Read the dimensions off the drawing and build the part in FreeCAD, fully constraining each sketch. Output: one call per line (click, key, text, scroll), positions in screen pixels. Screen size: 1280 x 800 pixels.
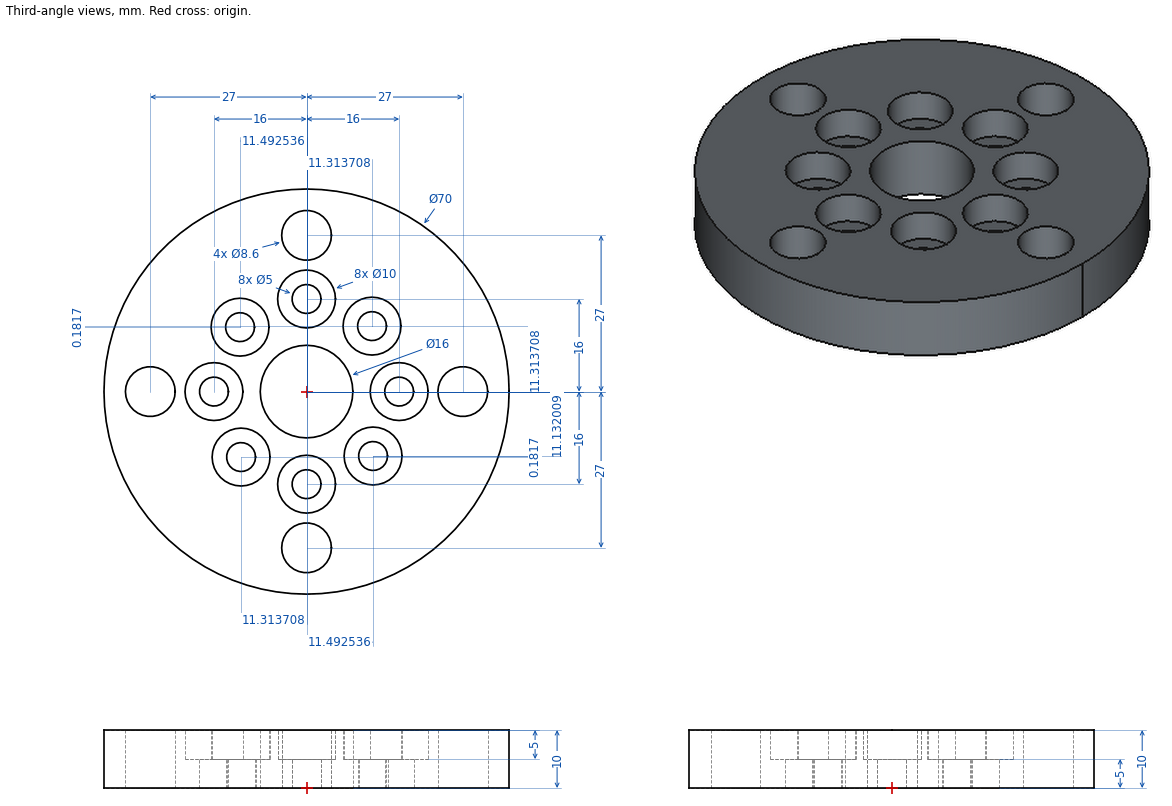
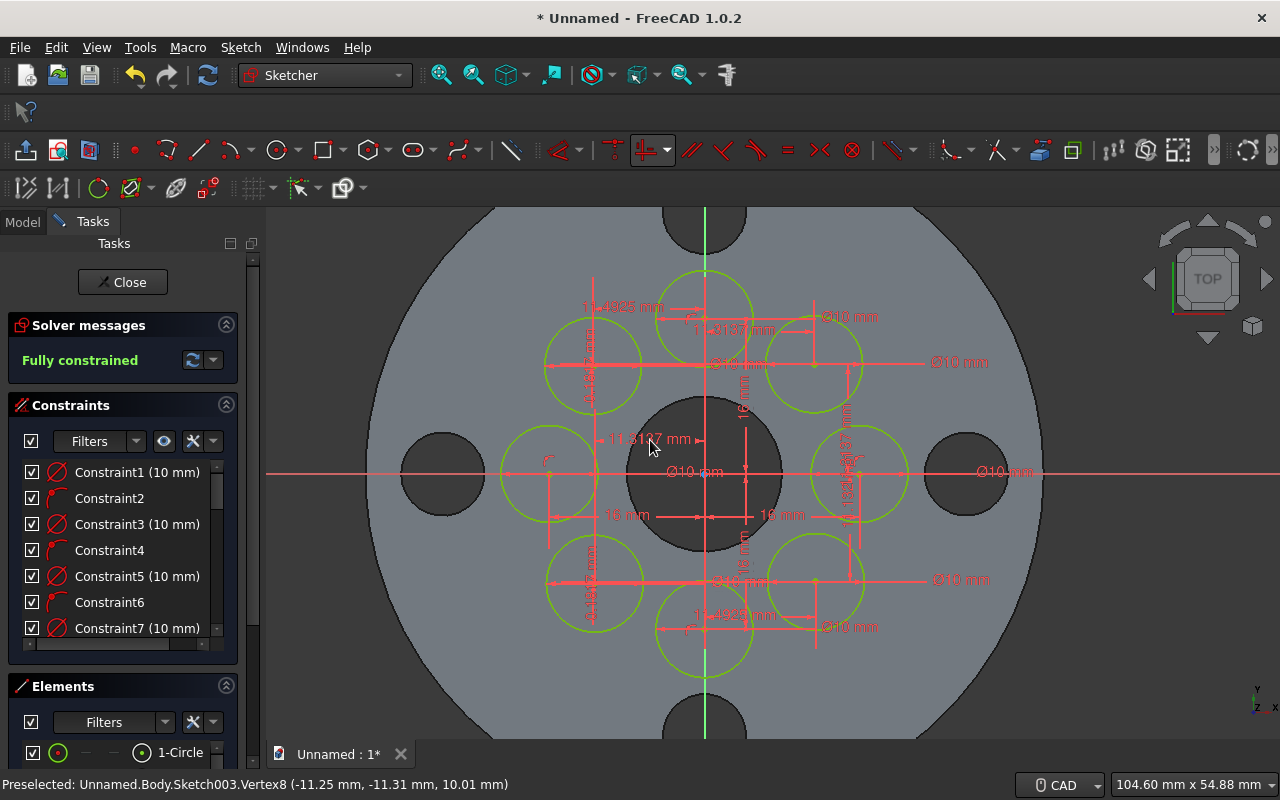
click(123, 282)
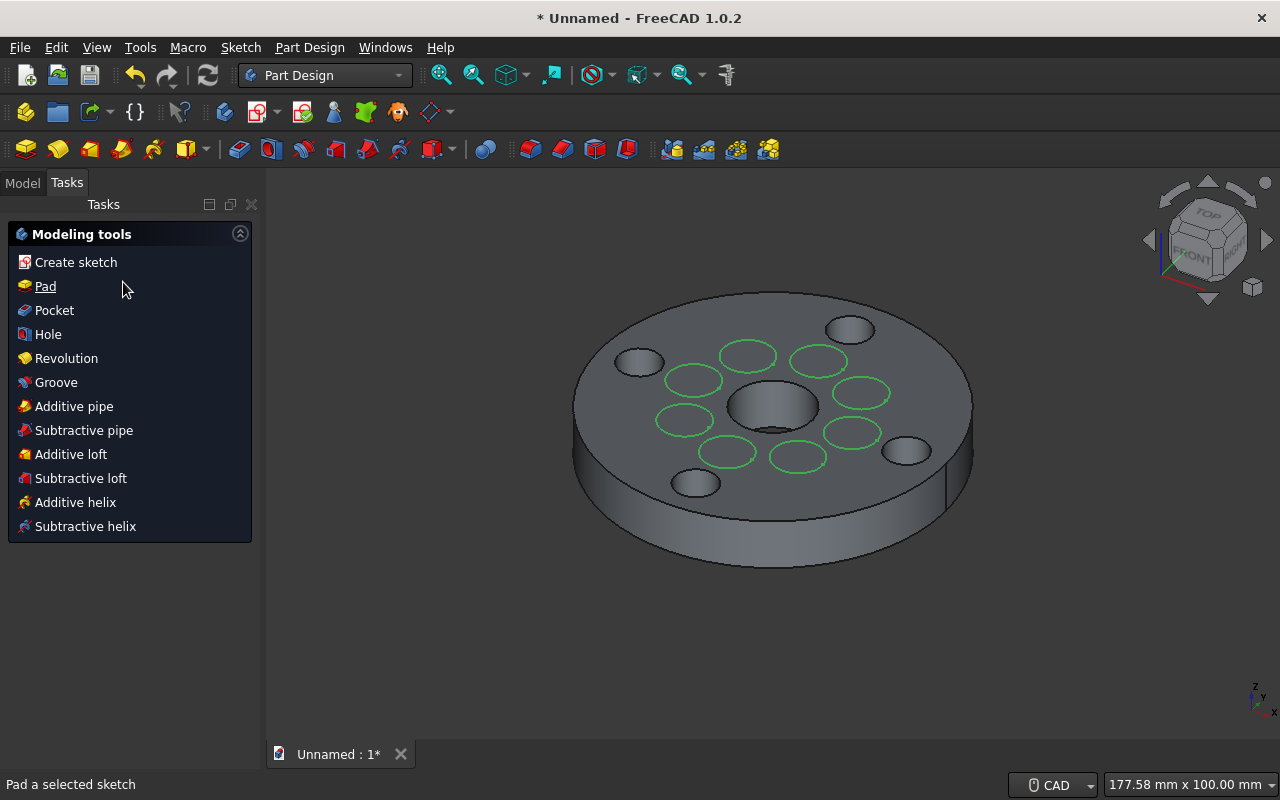
click(240, 150)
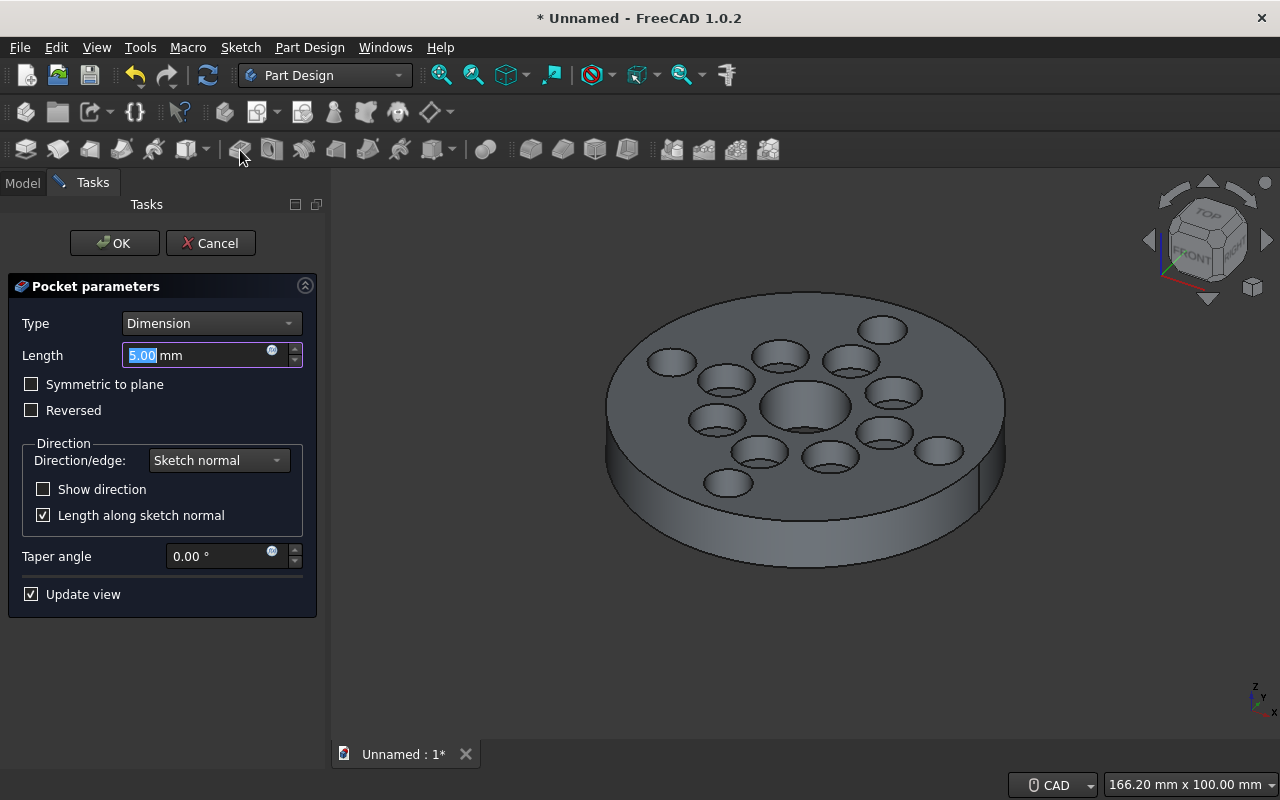
text(5)
key(Tab)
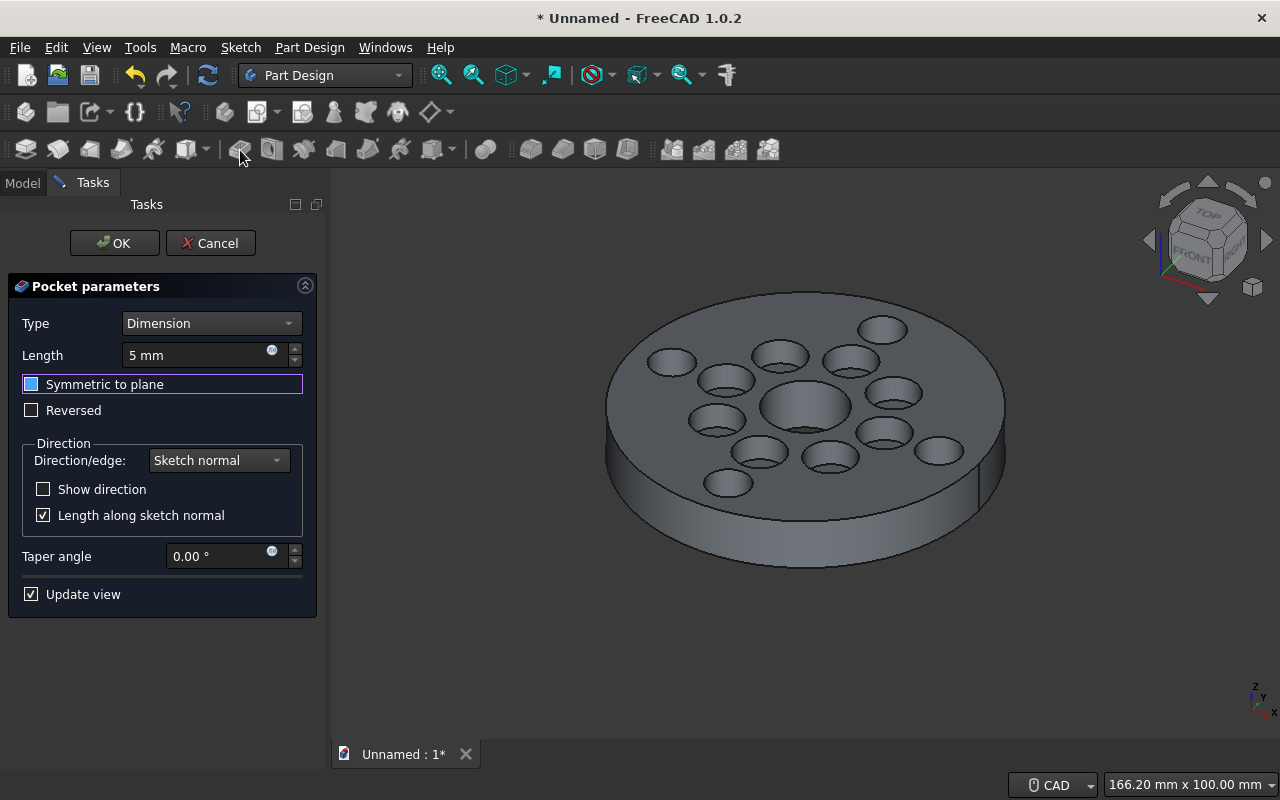
click(115, 243)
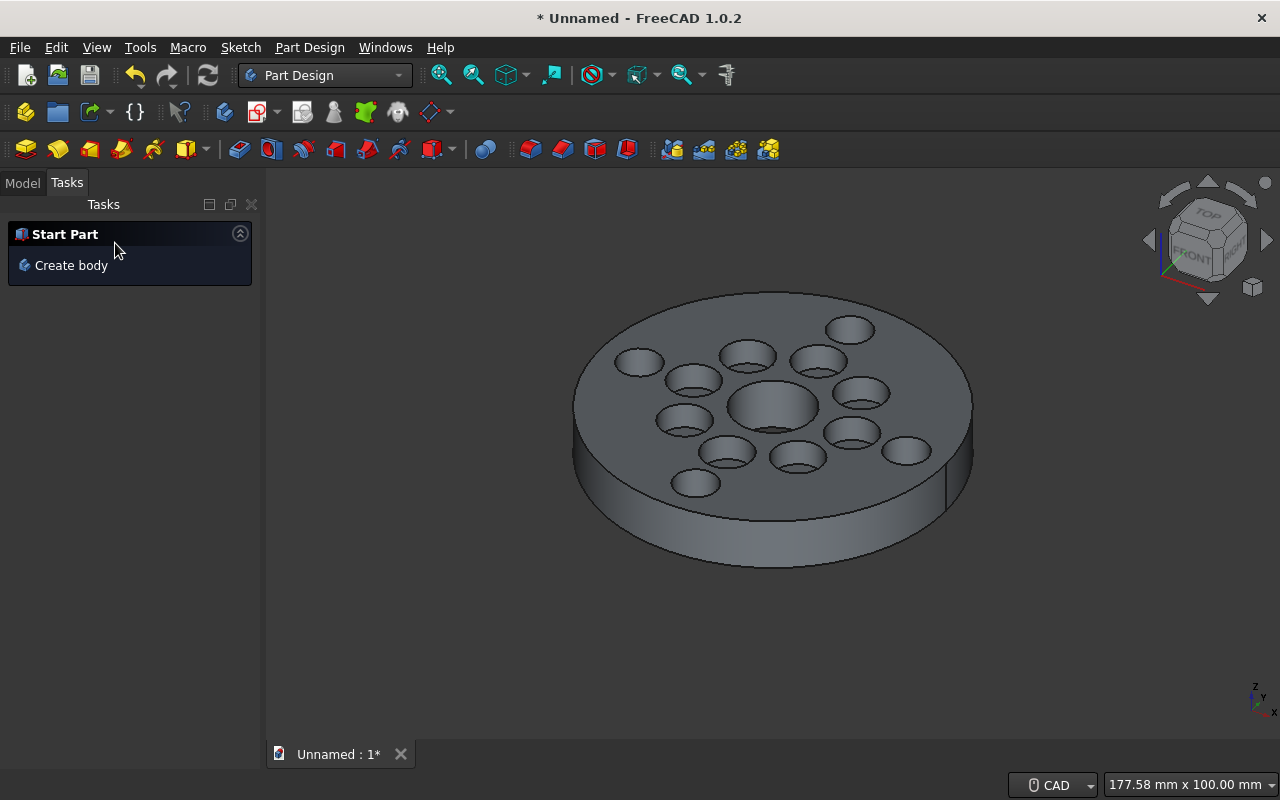
key(0)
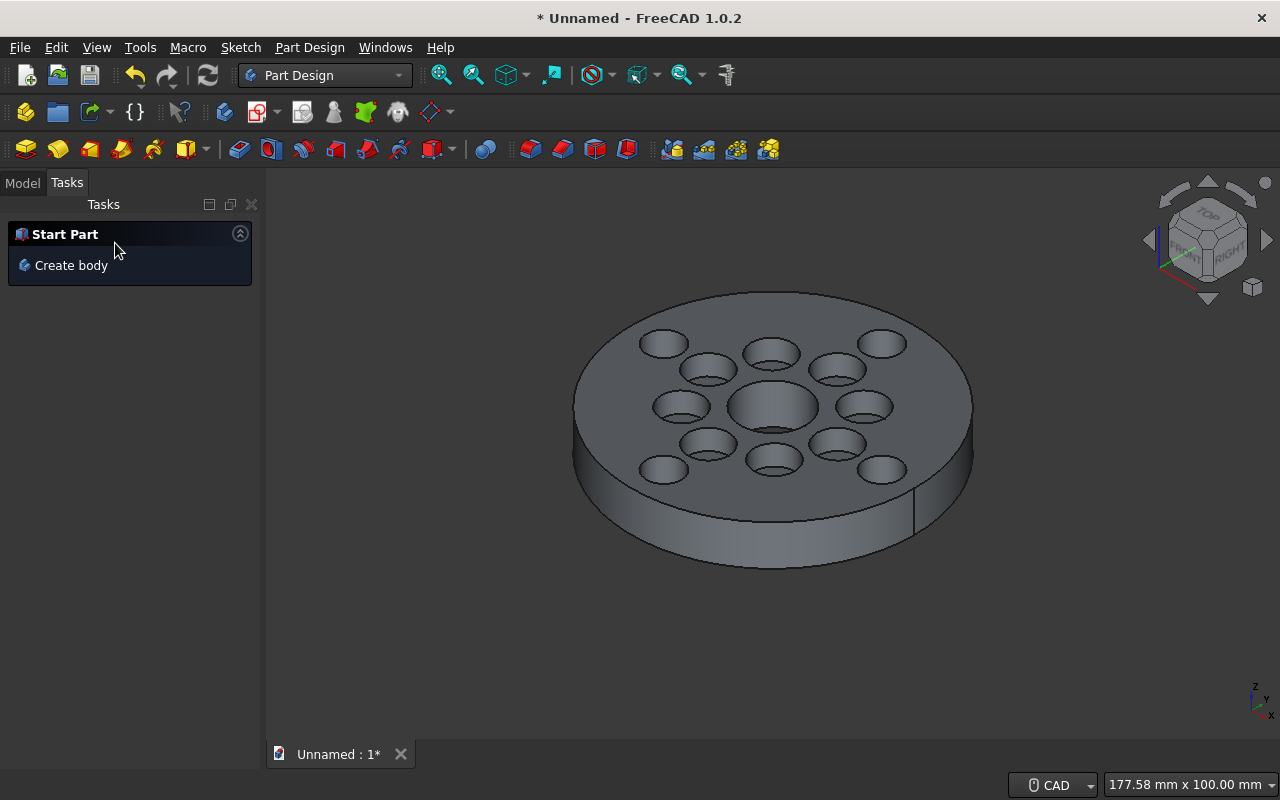
key(2)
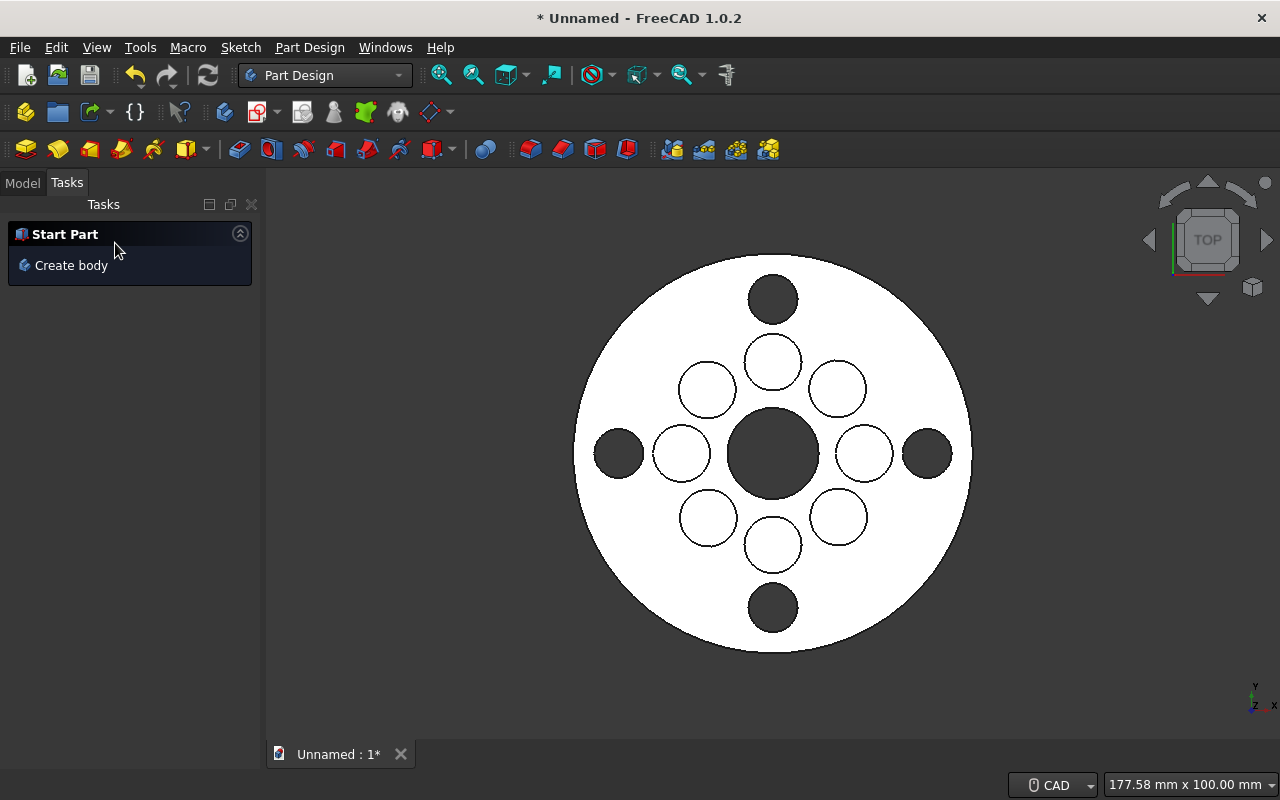
click(839, 516)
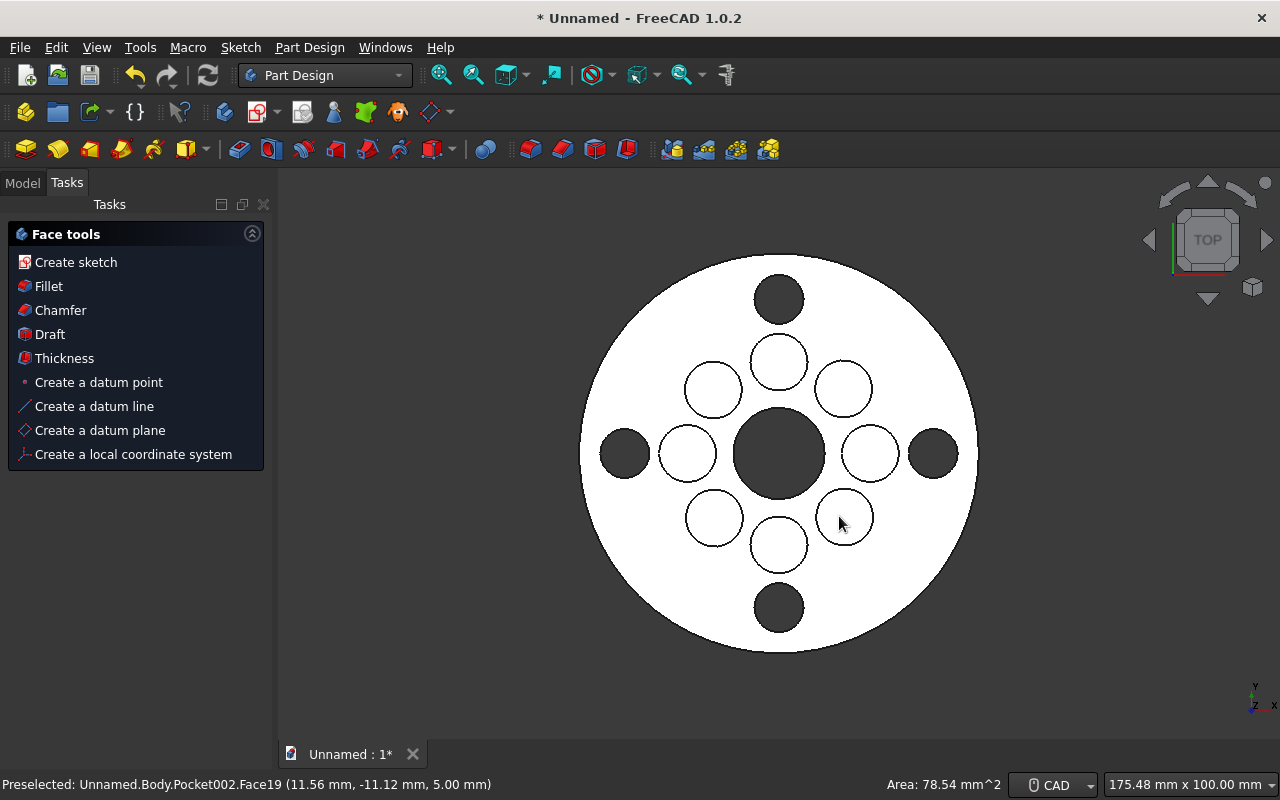
click(258, 112)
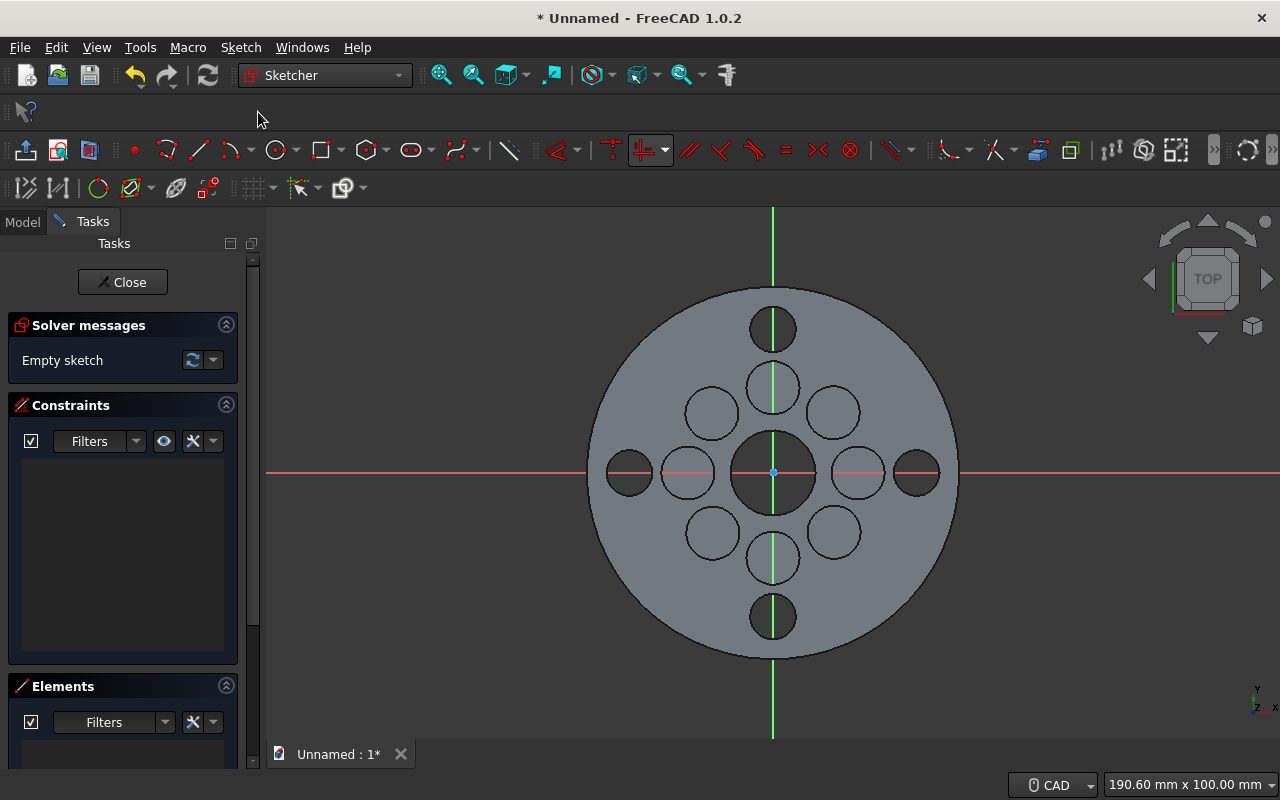
scroll(856, 473, up, 3)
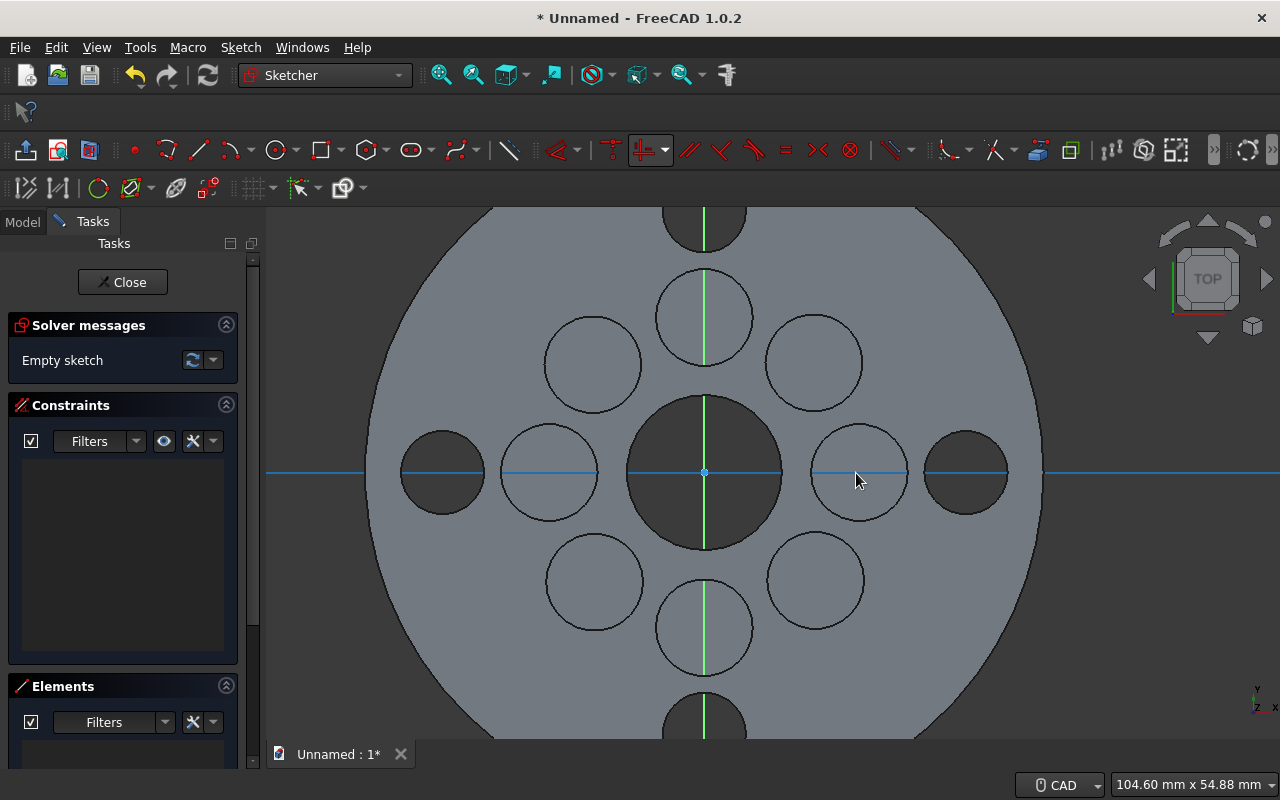
click(276, 150)